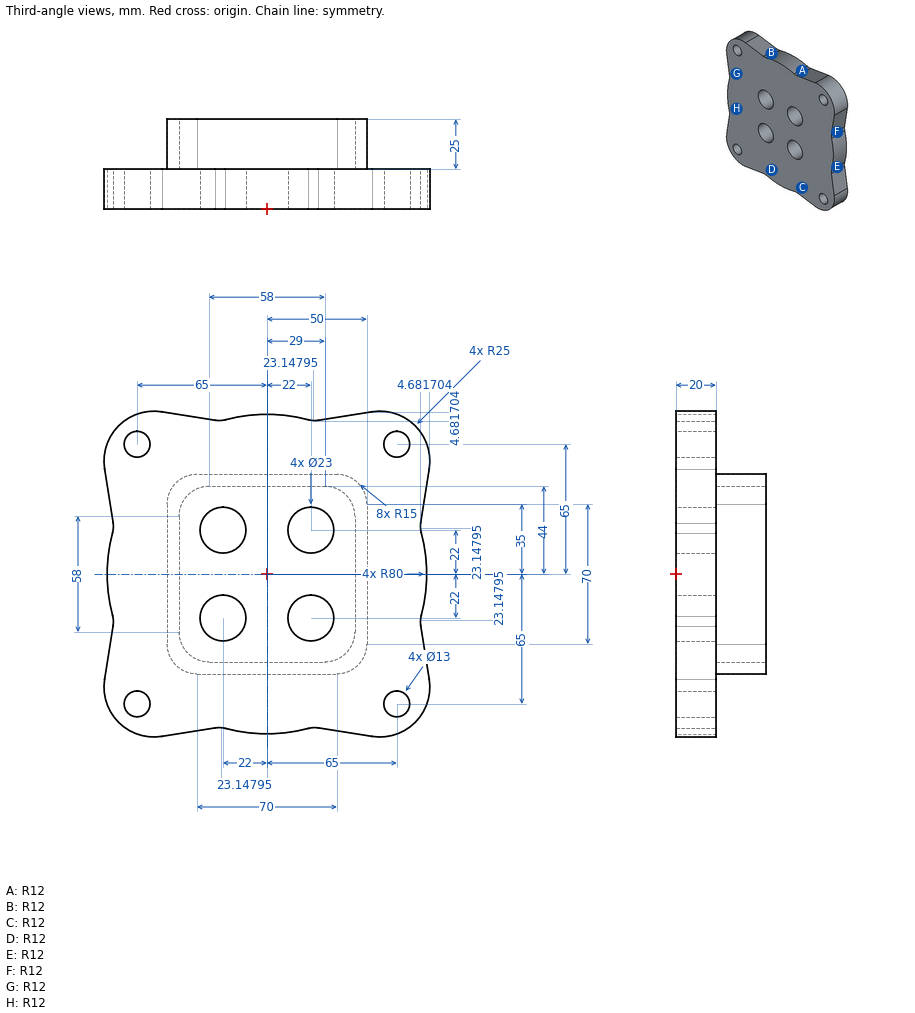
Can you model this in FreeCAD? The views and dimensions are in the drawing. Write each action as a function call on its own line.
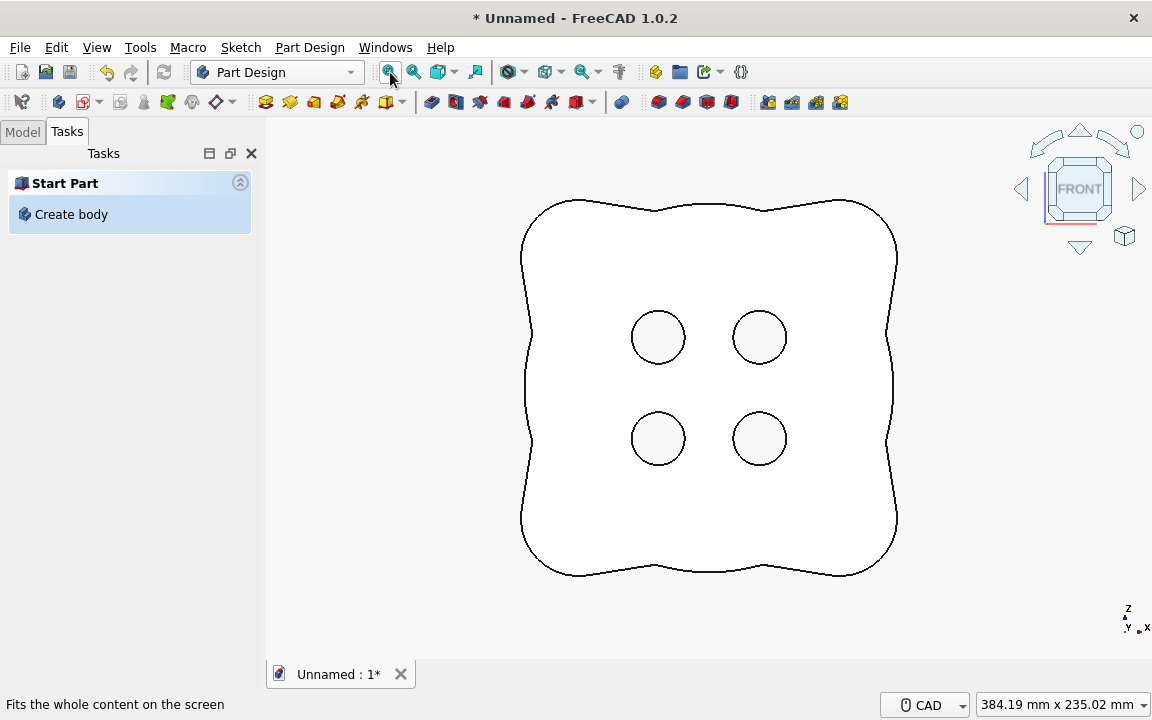
key(3)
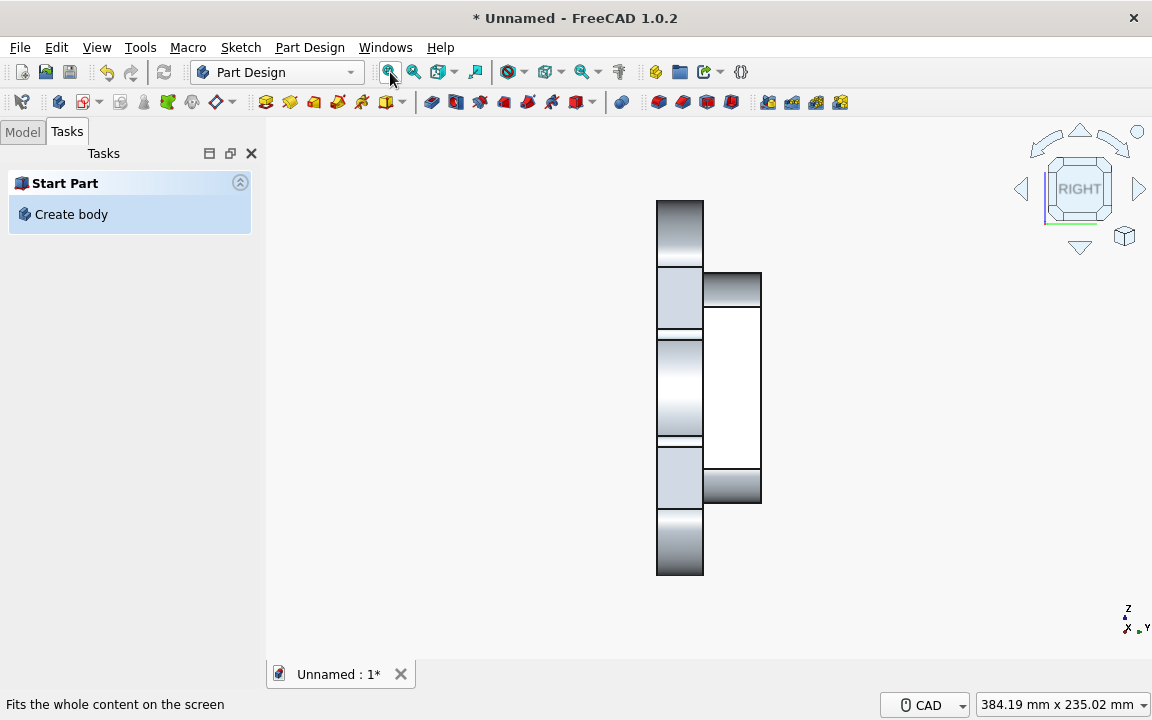
key(5)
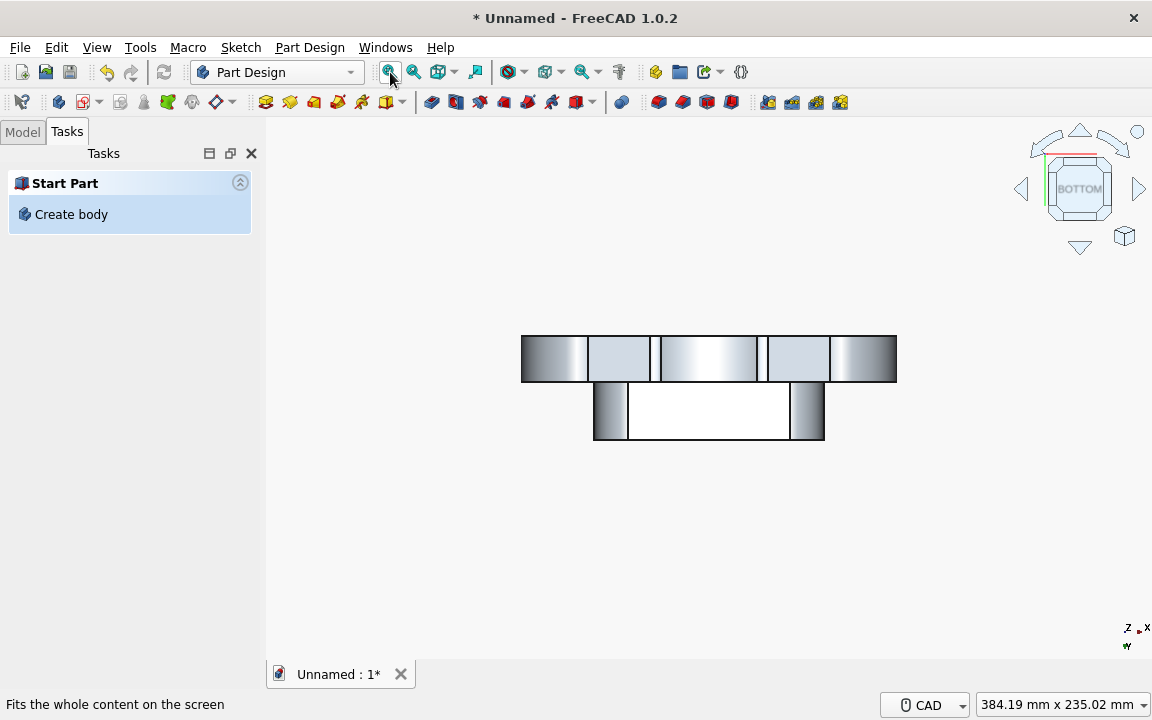
click(390, 72)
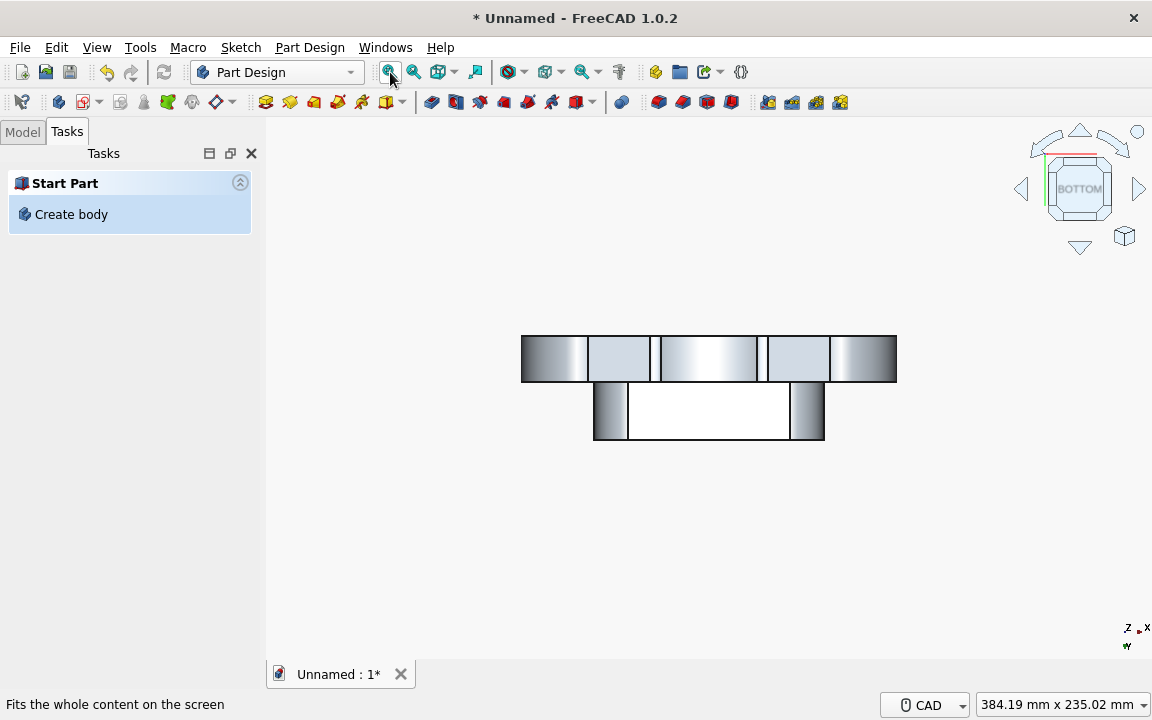
key(4)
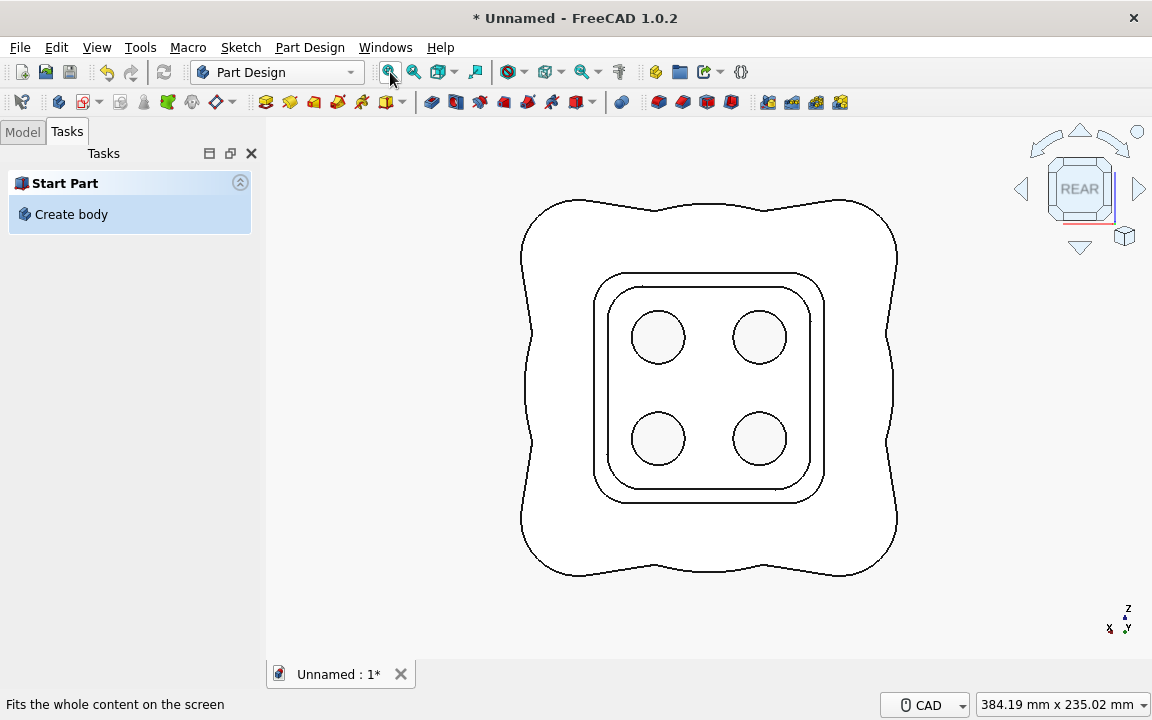
key(6)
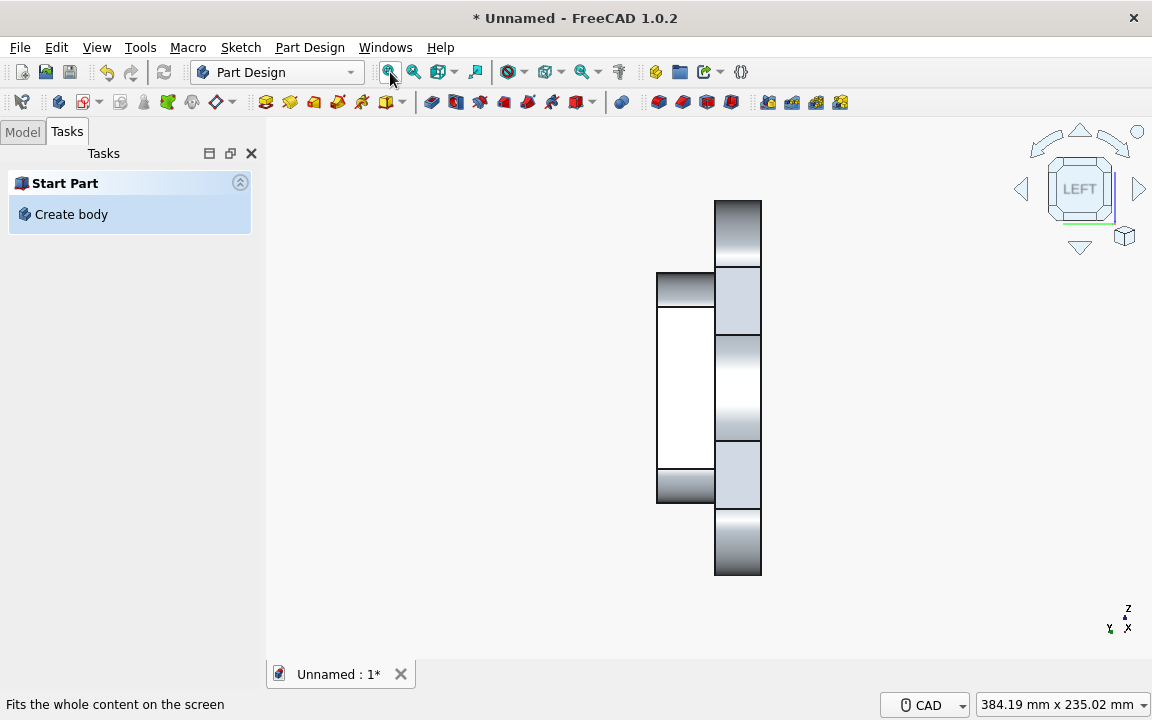
key(v)
key(3)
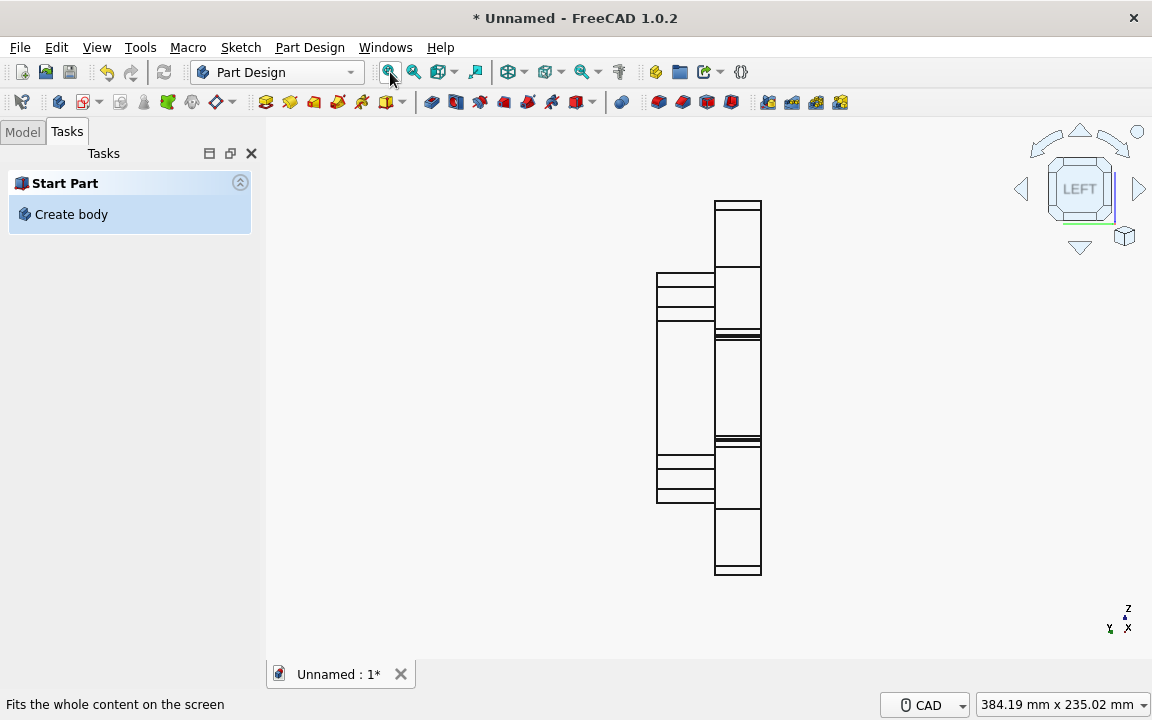
key(0)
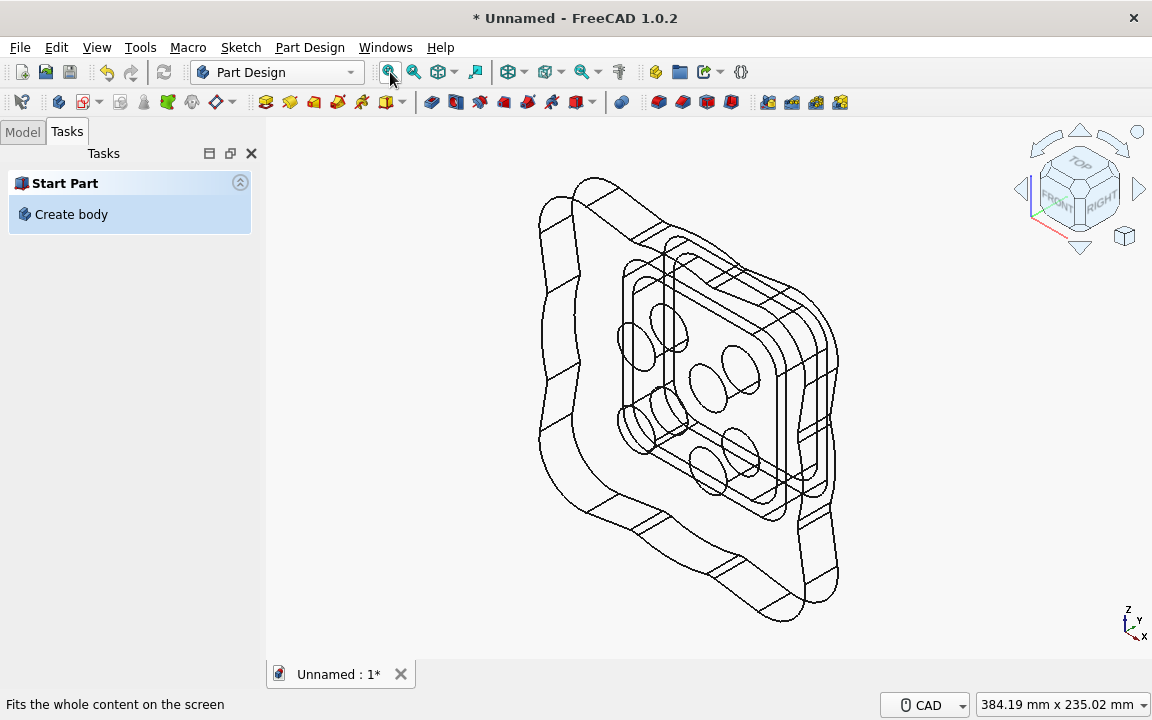
click(564, 283)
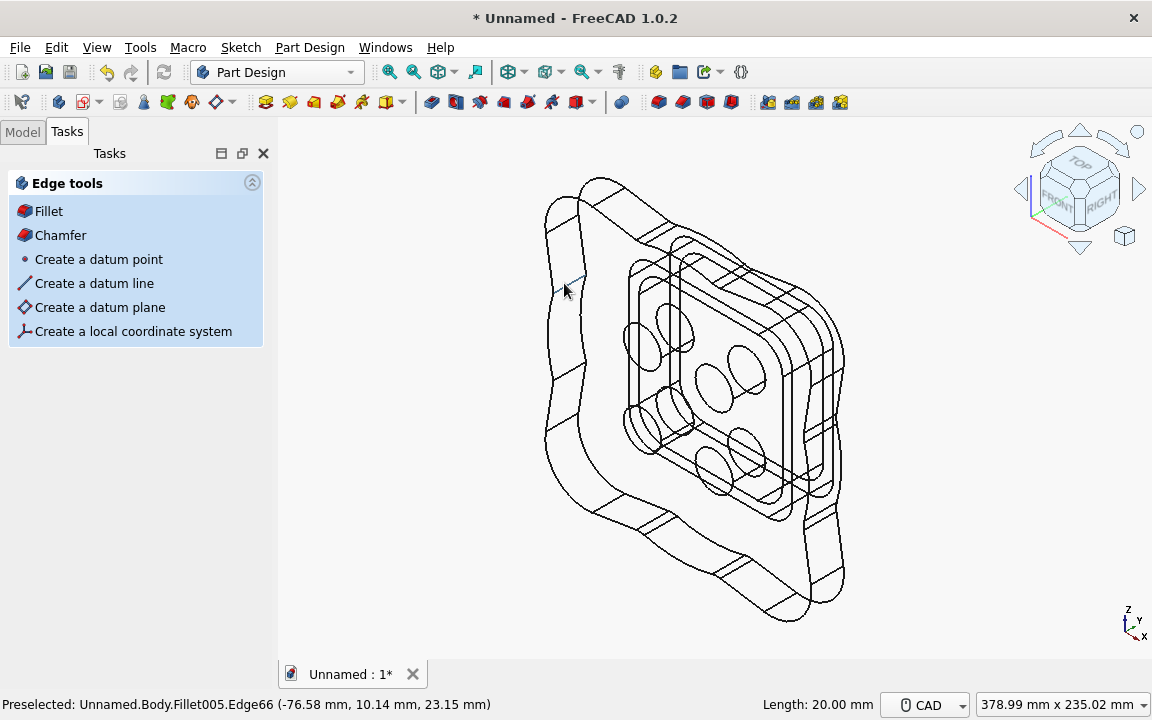
key(v)
key(1)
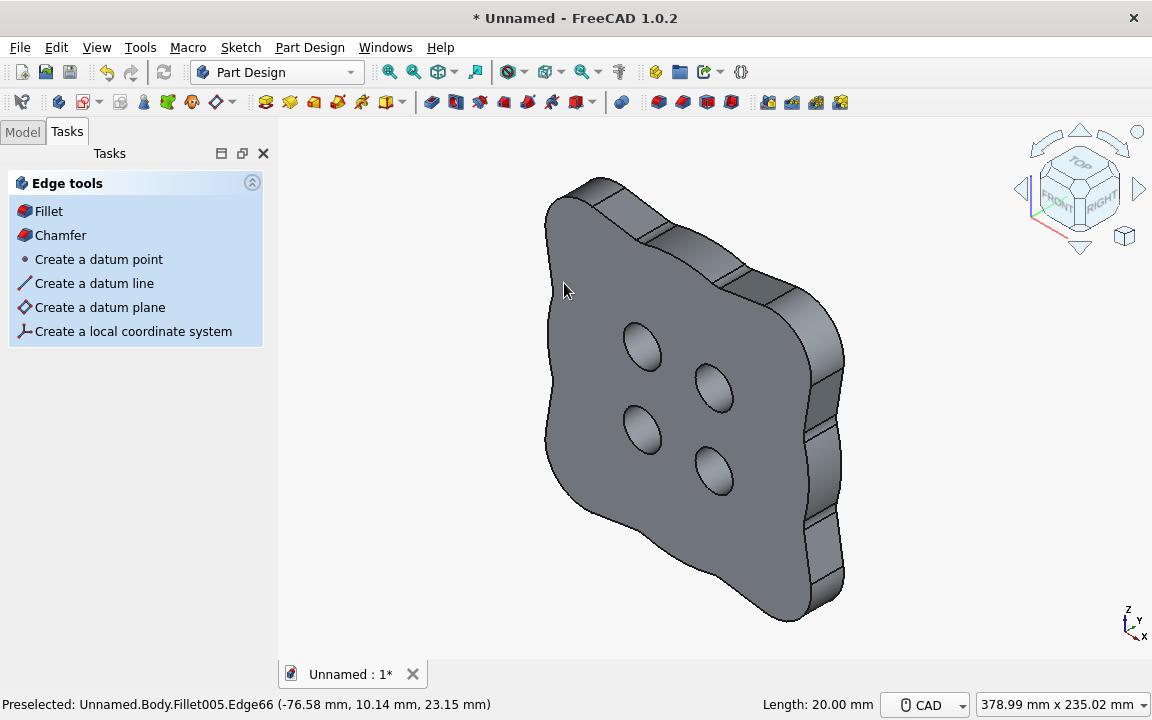
click(660, 102)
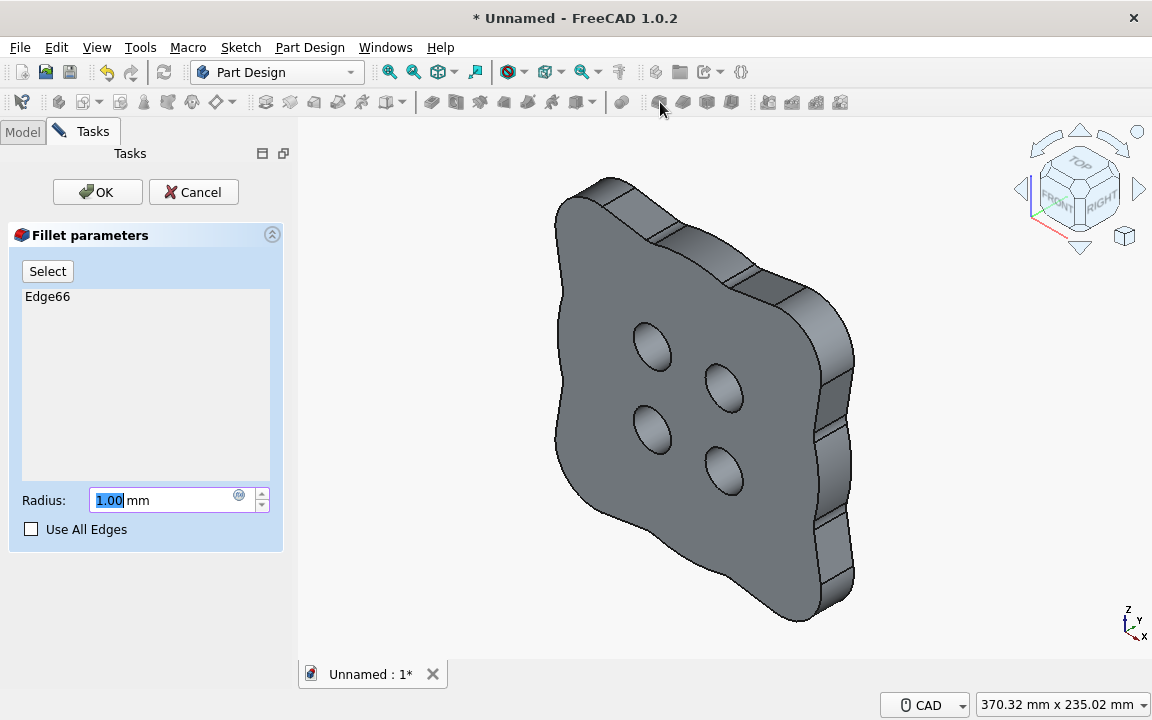
text(12)
key(Tab)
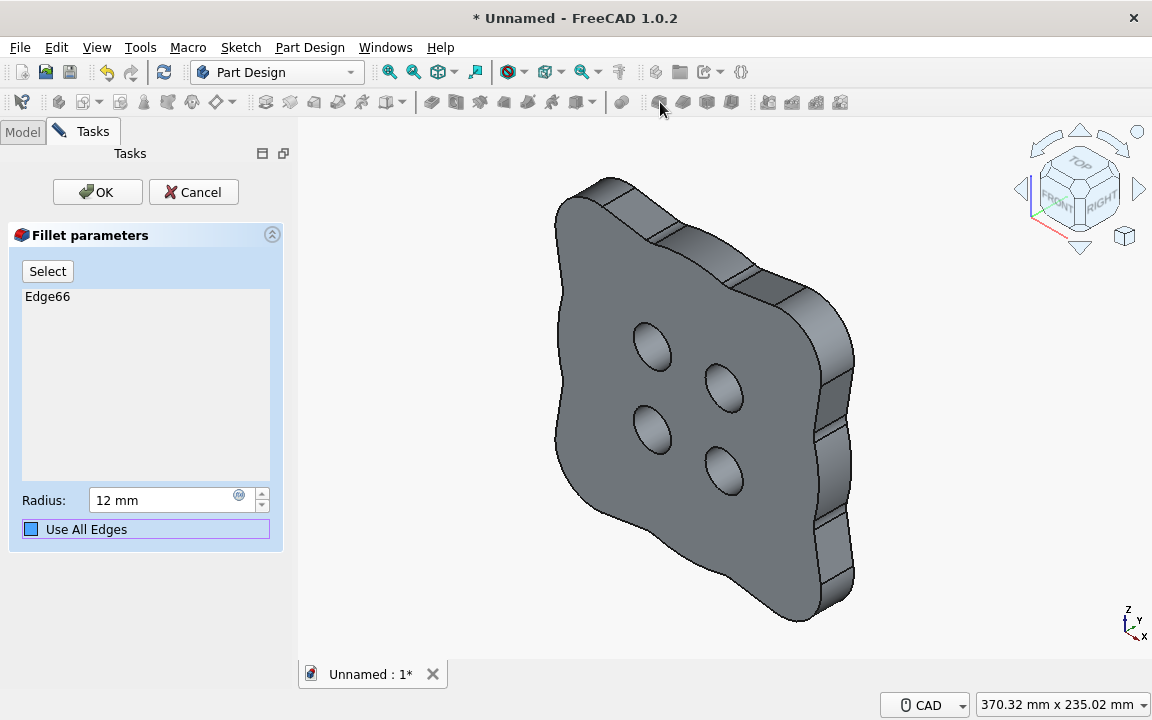
click(98, 192)